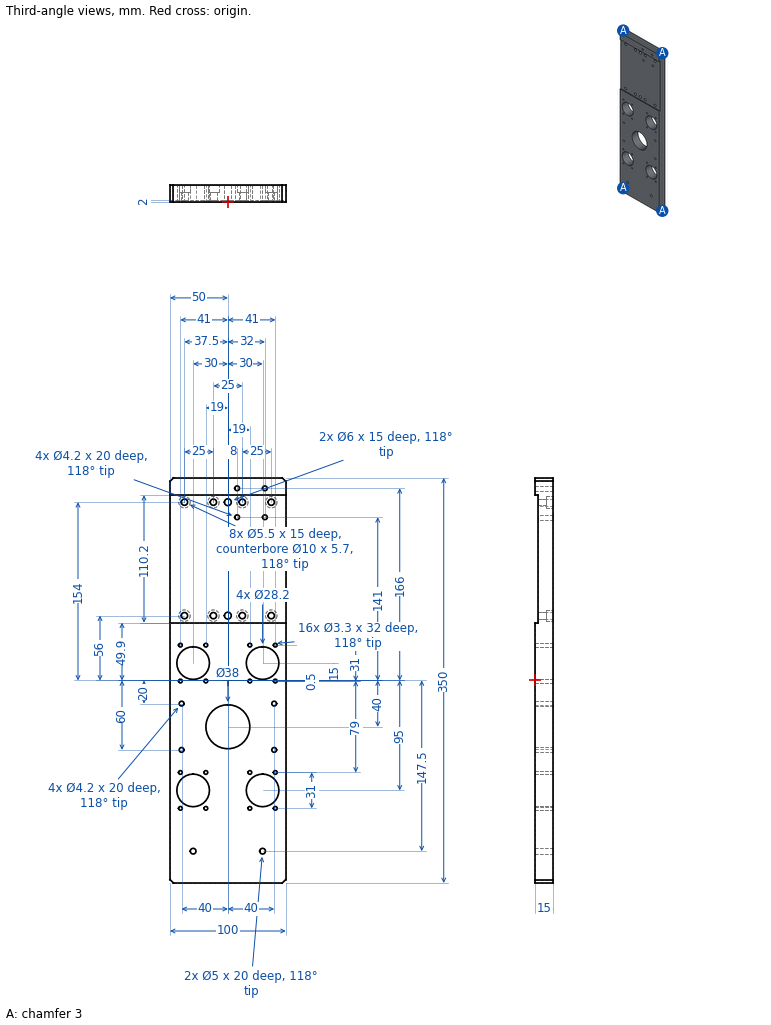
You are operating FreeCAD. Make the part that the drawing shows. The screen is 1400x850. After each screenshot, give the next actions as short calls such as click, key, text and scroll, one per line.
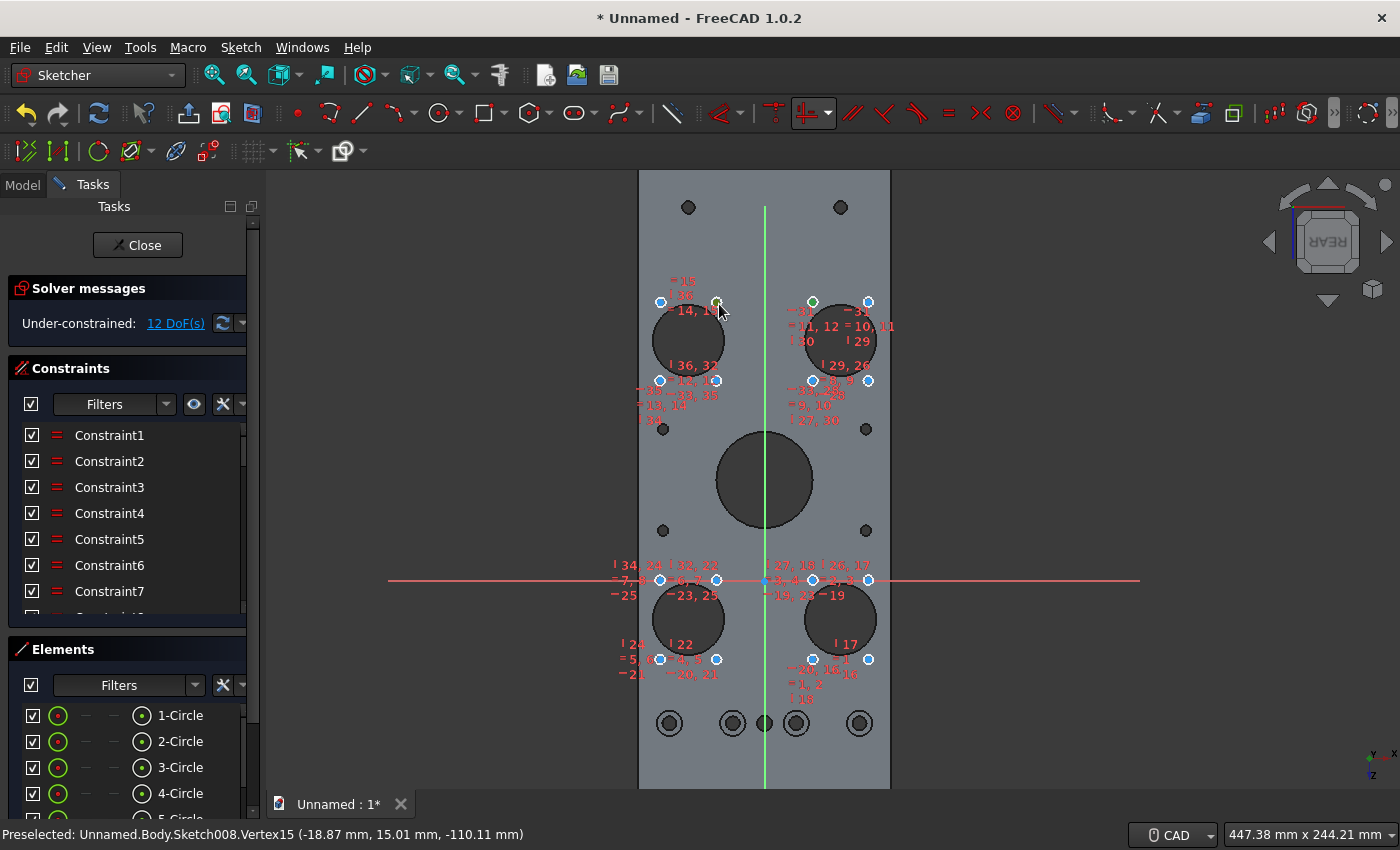
click(830, 114)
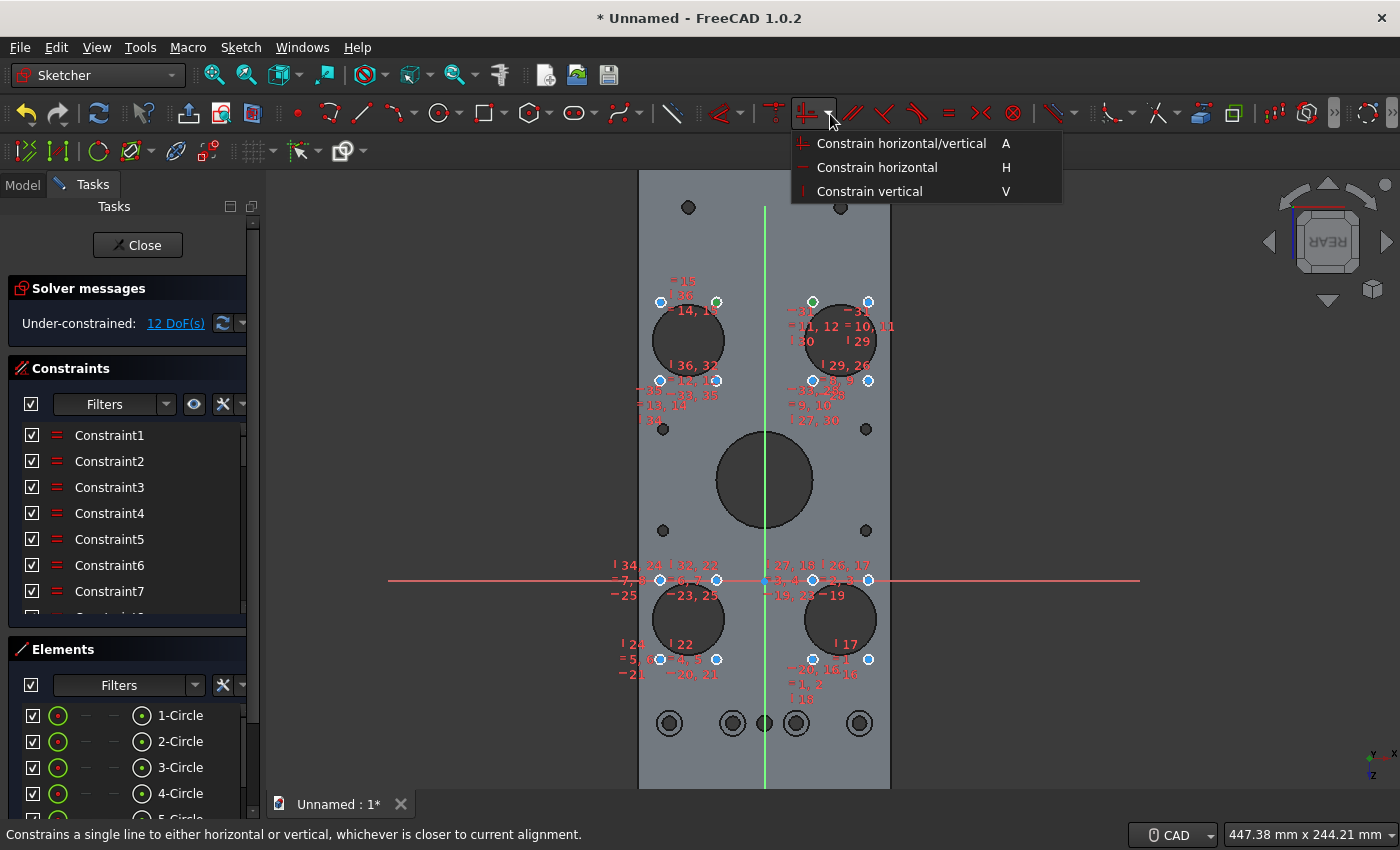
click(927, 167)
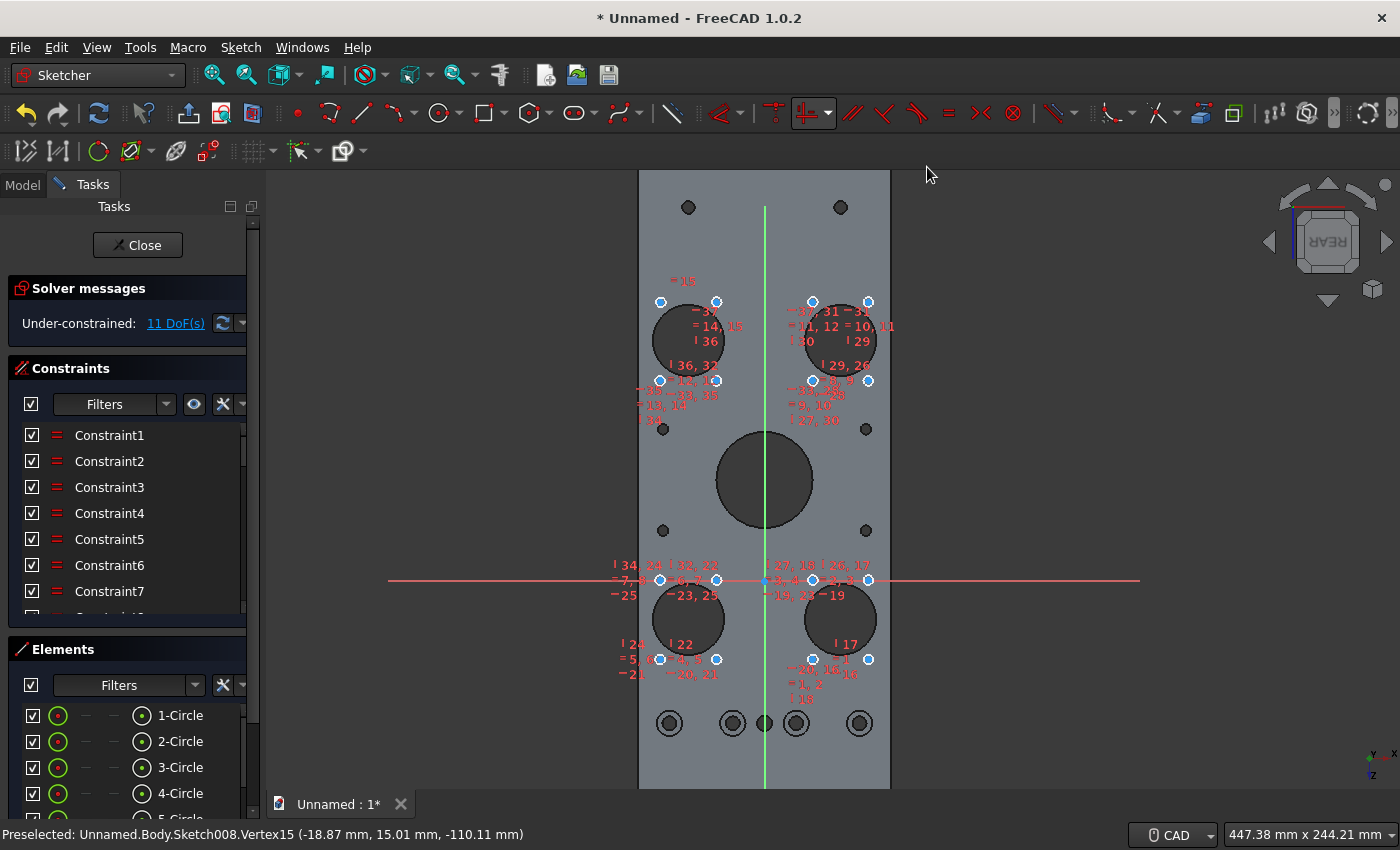
click(660, 381)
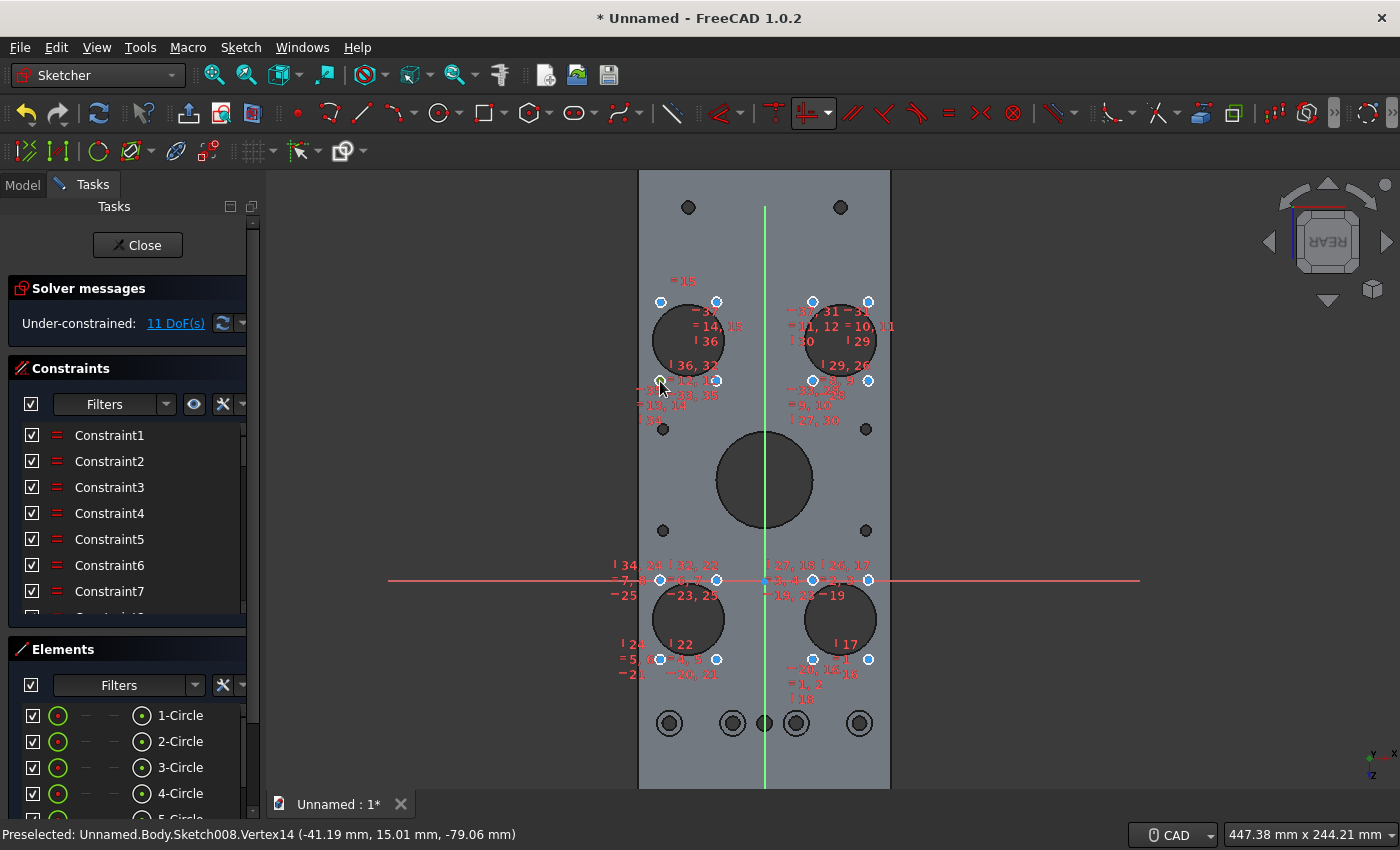
click(661, 302)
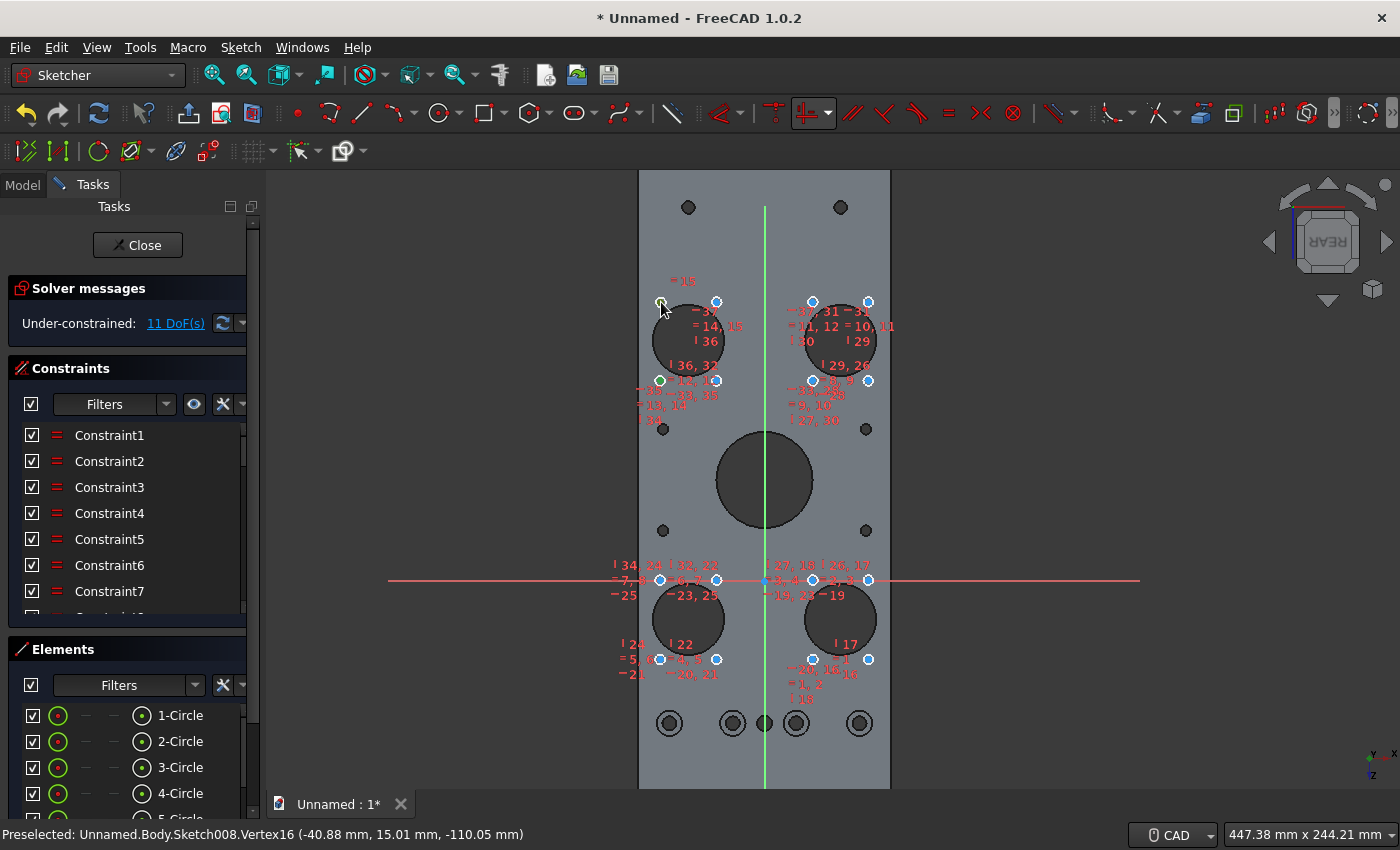
key(v)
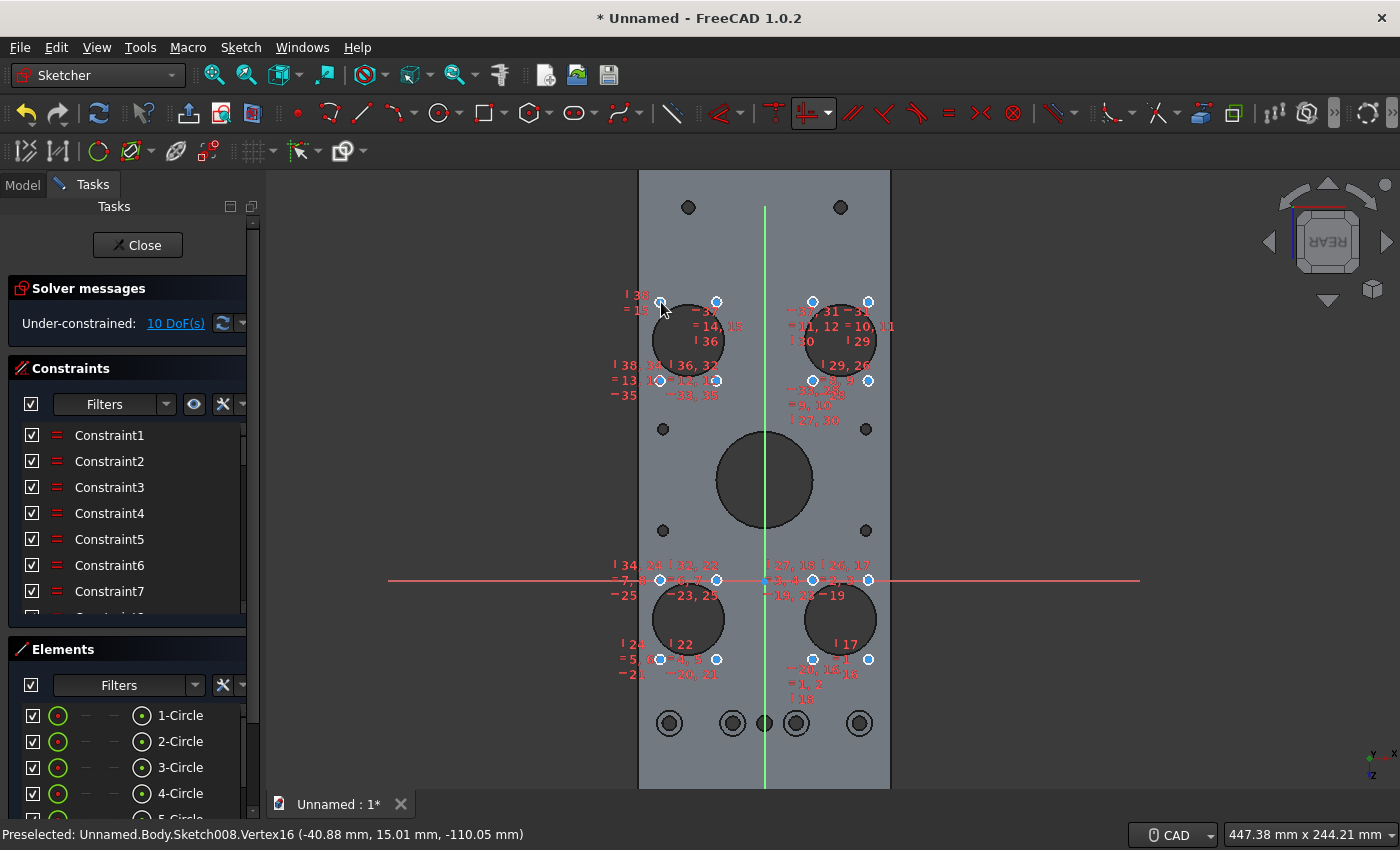
click(717, 302)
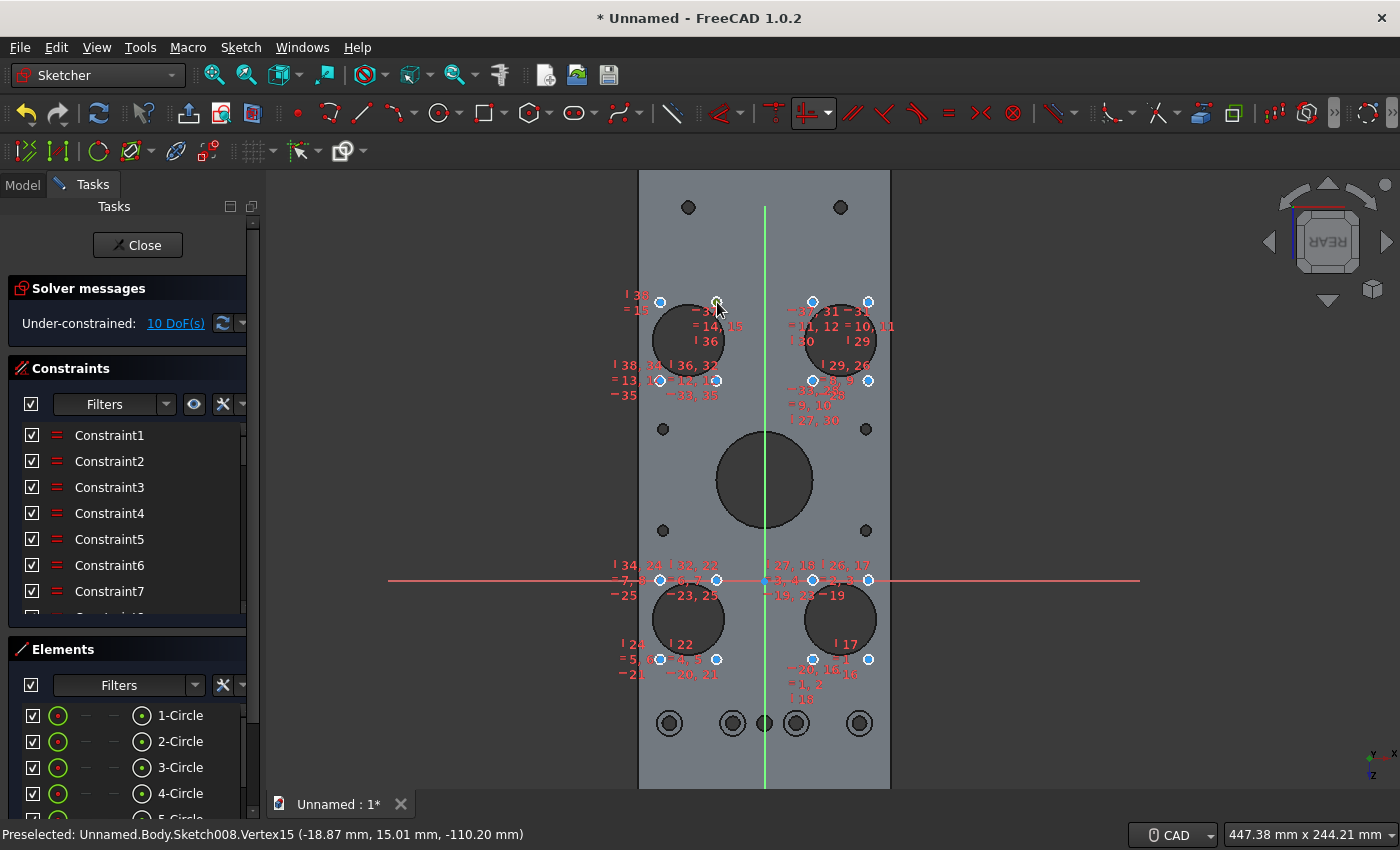
click(660, 302)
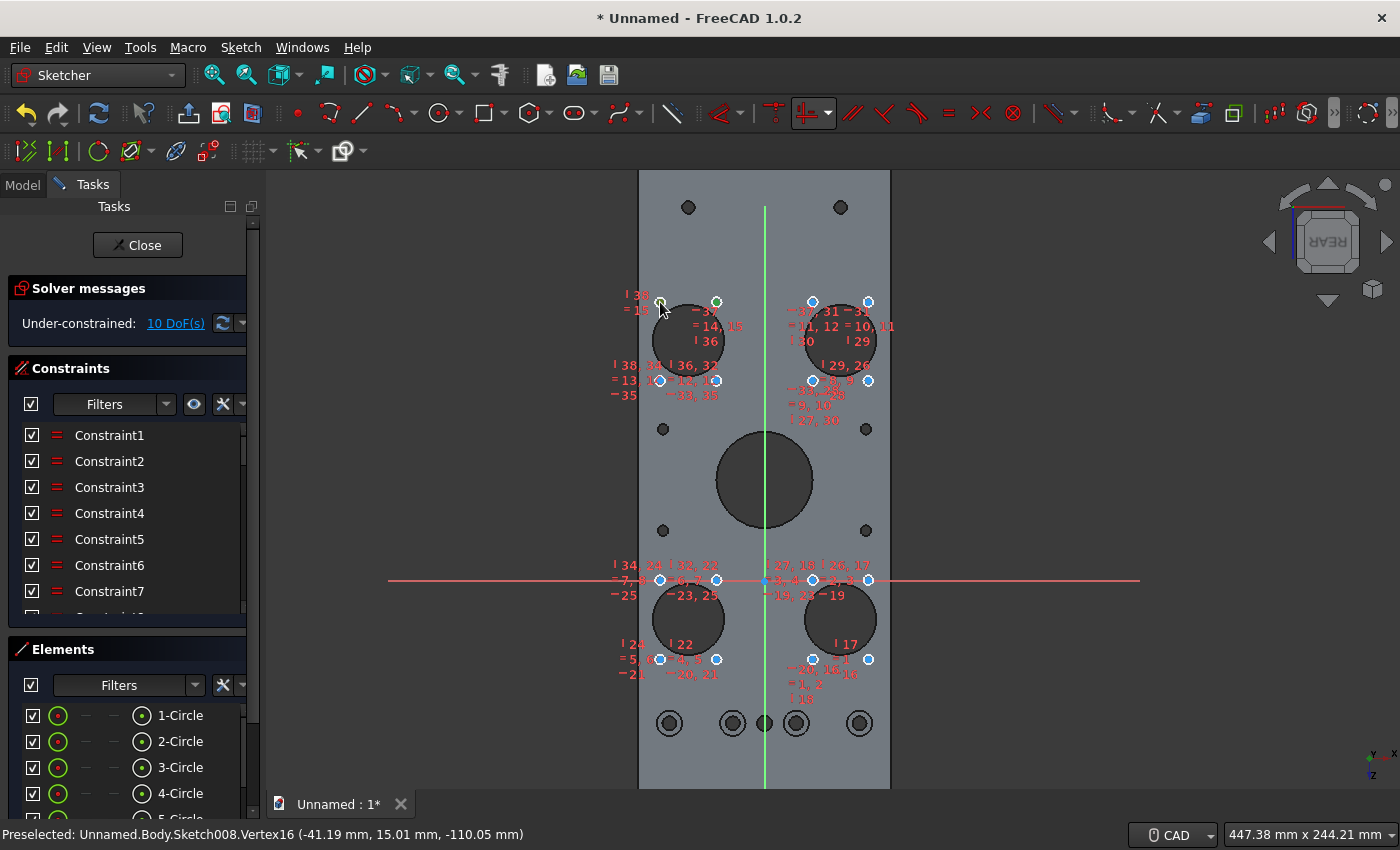
key(h)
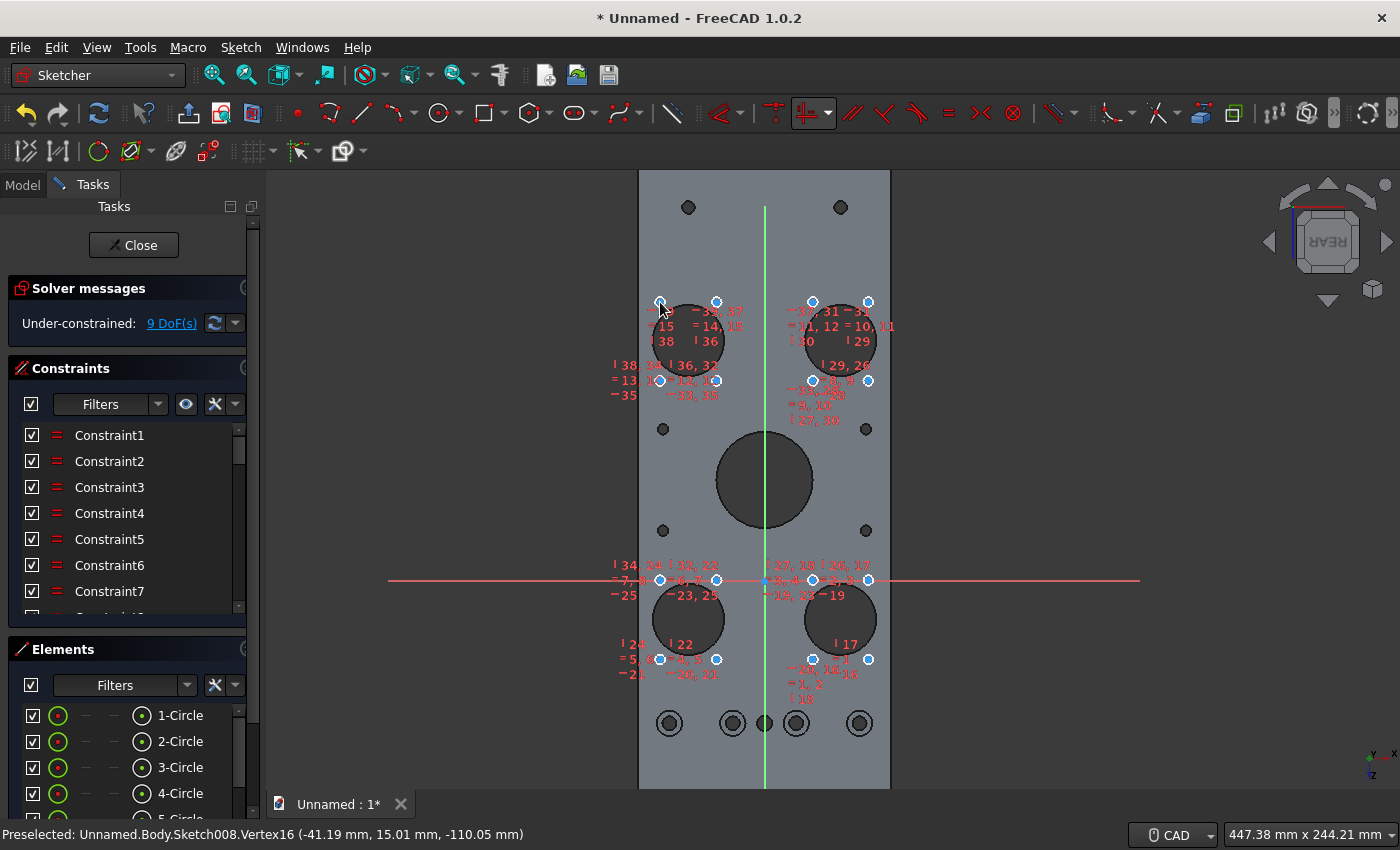
key(d)